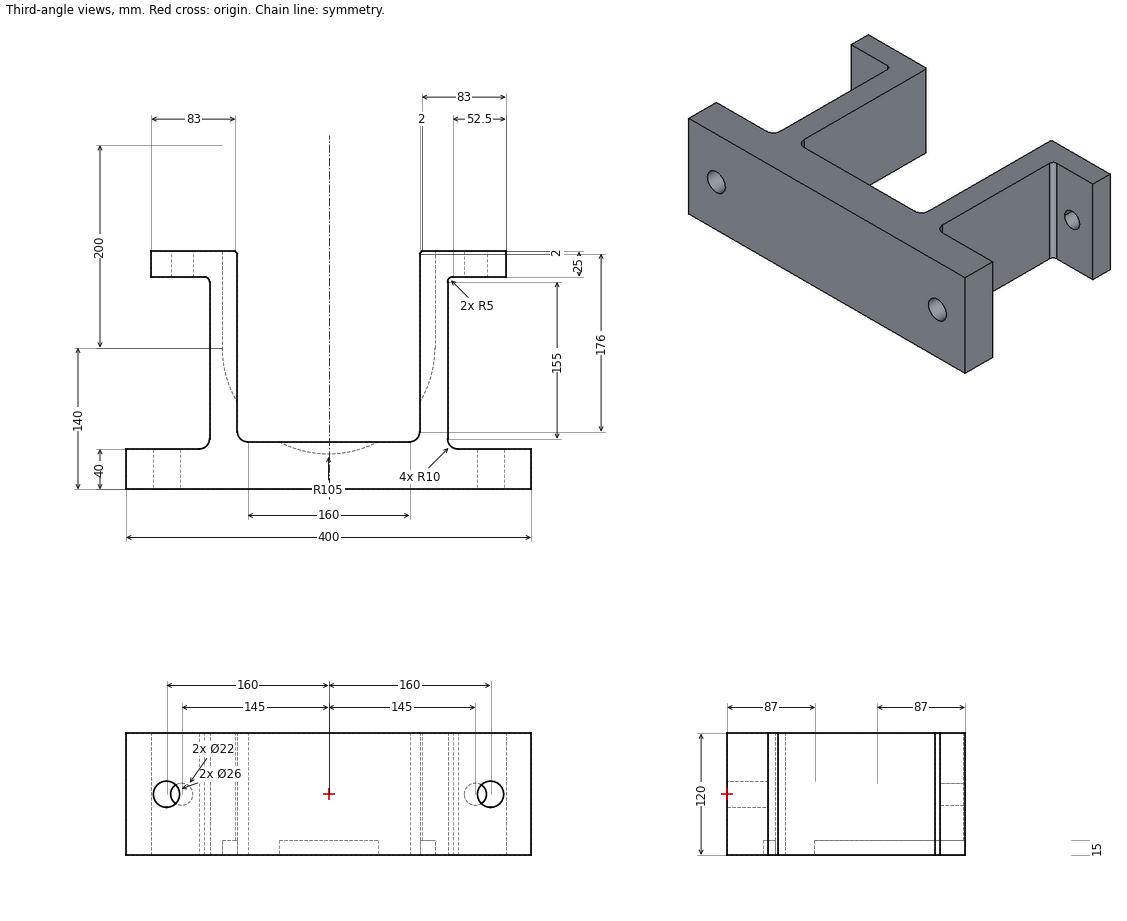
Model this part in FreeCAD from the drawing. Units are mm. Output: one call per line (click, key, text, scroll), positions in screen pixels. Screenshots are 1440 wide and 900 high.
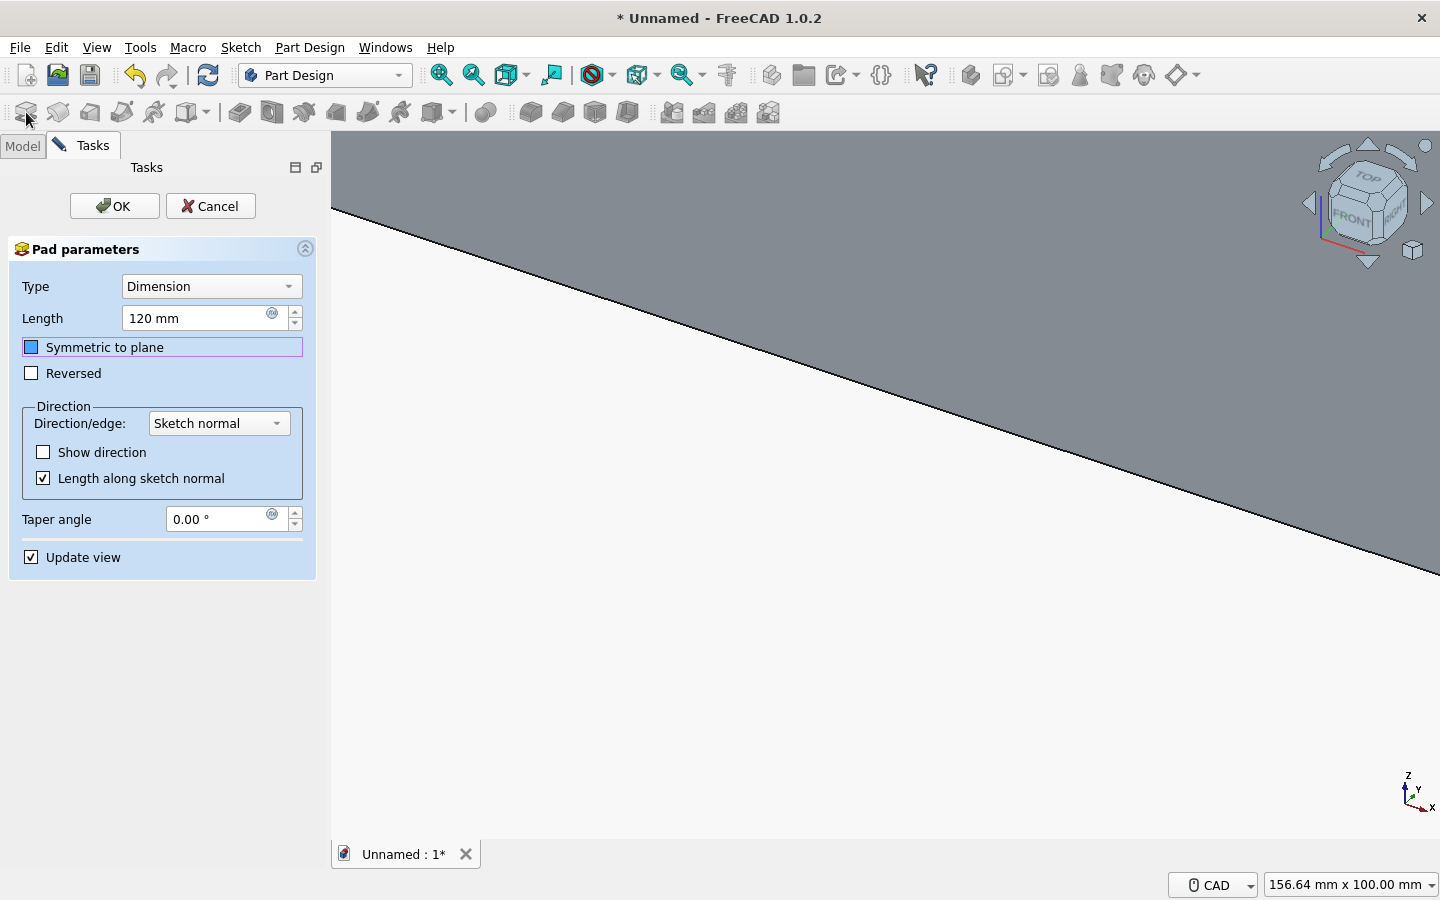
click(30, 347)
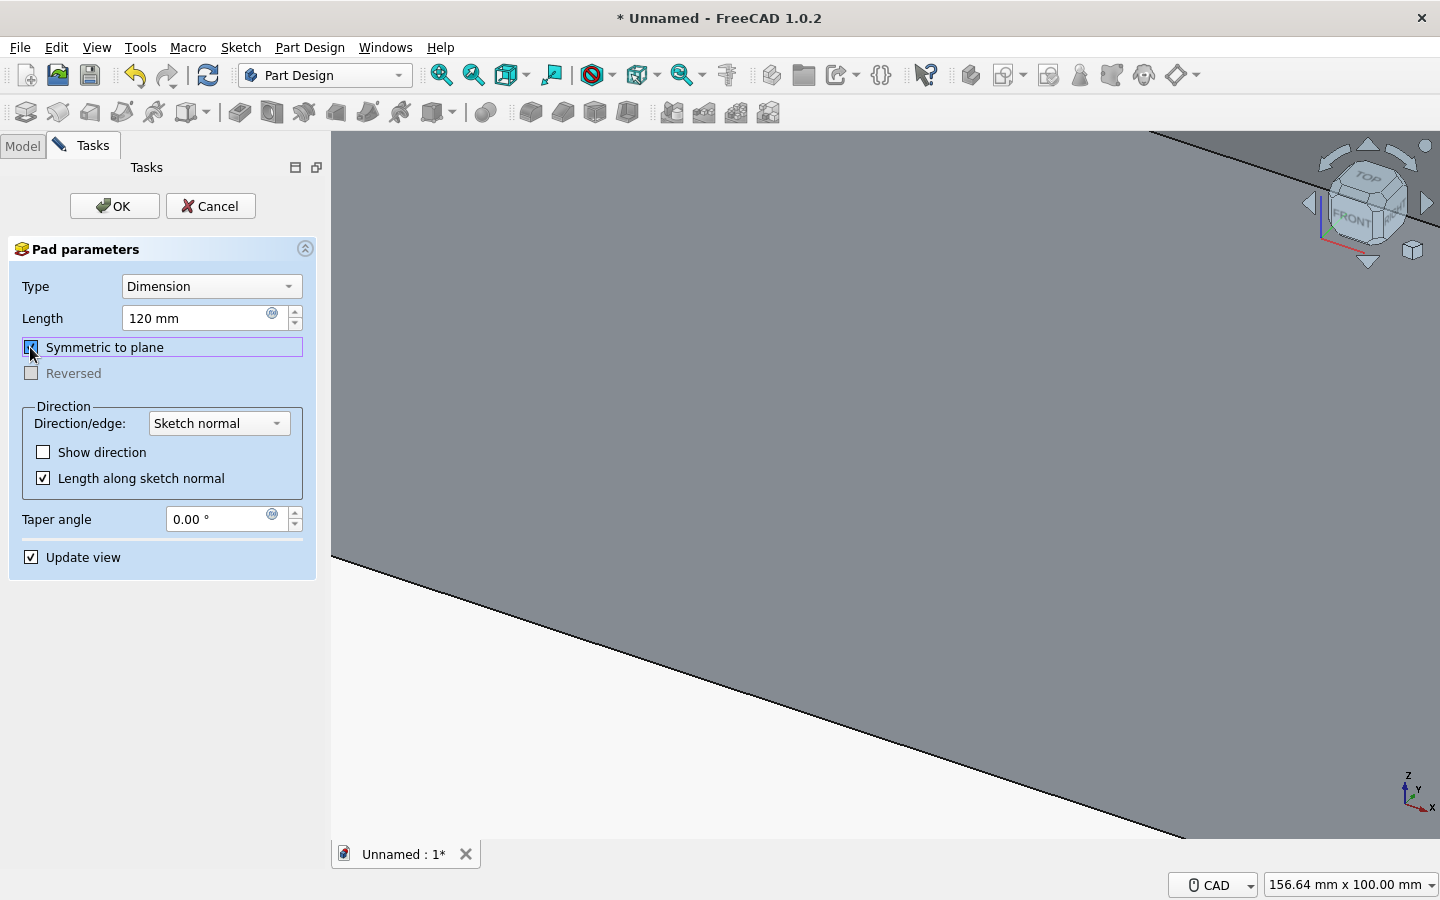
click(115, 206)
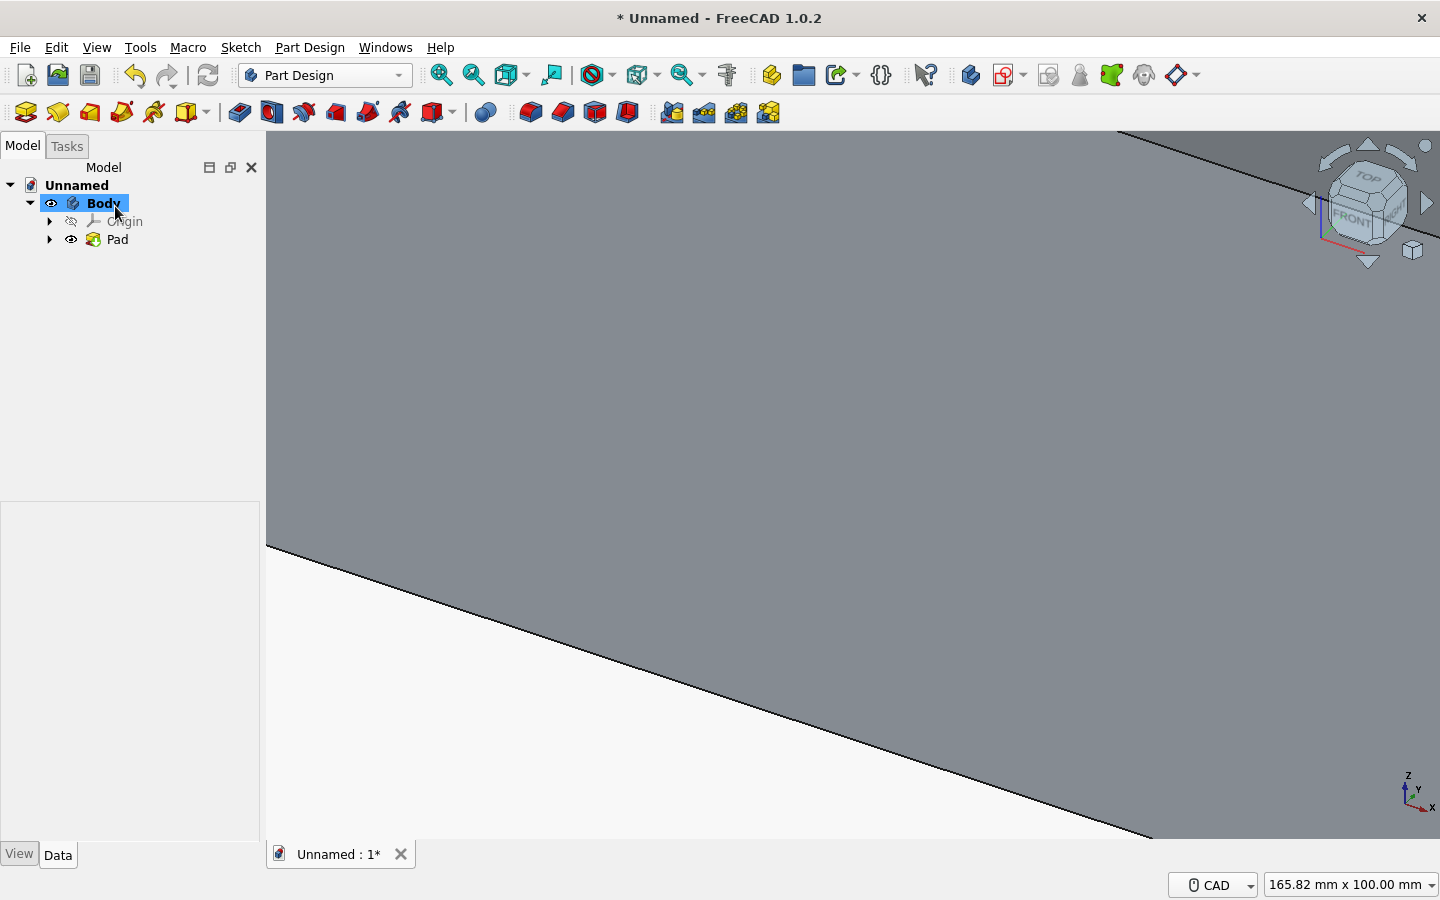
click(442, 76)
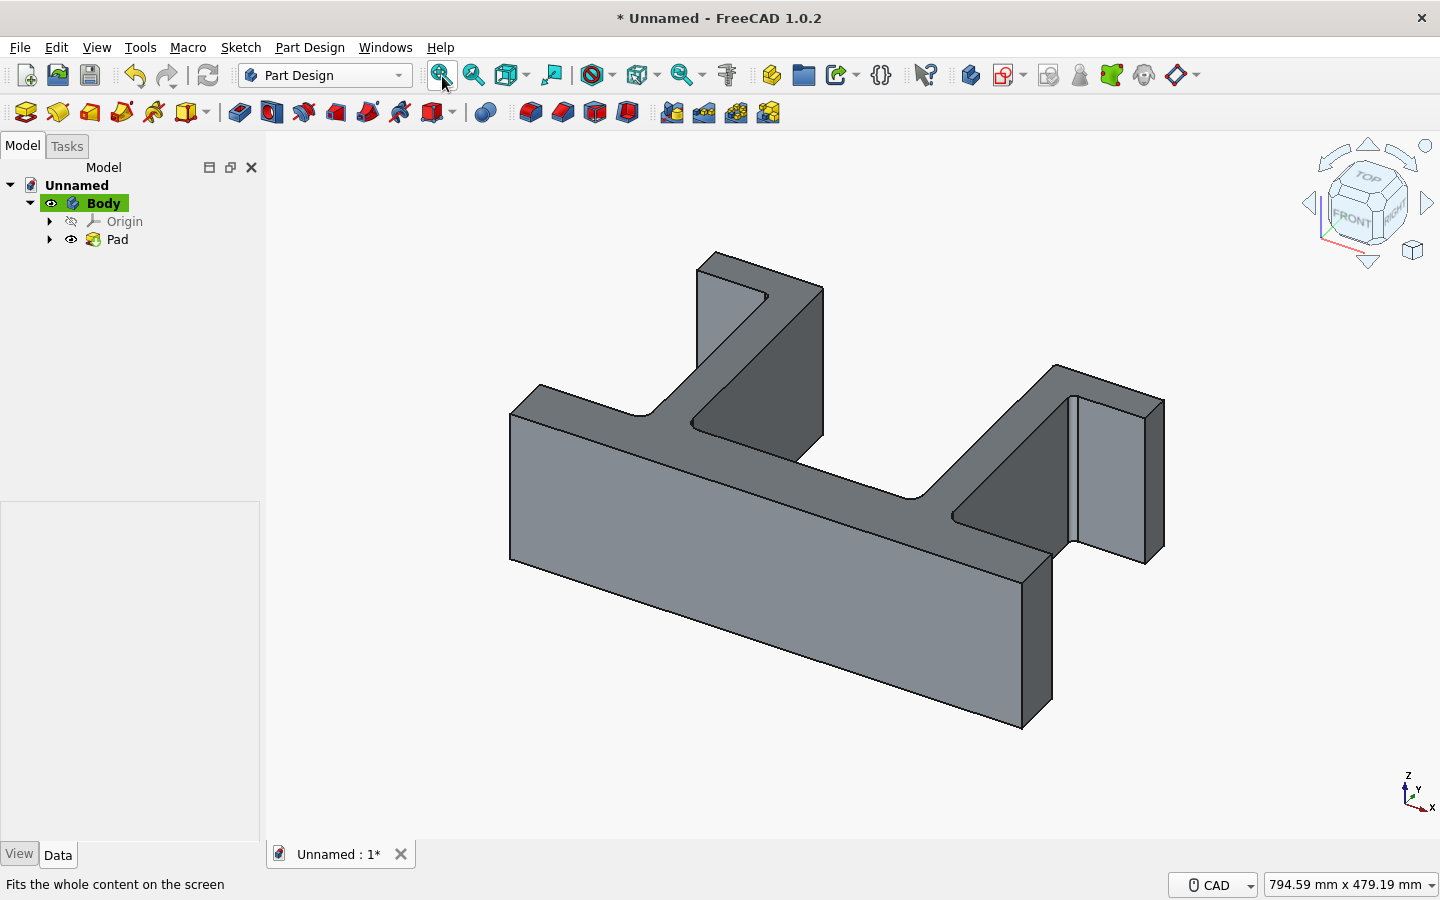
click(1004, 76)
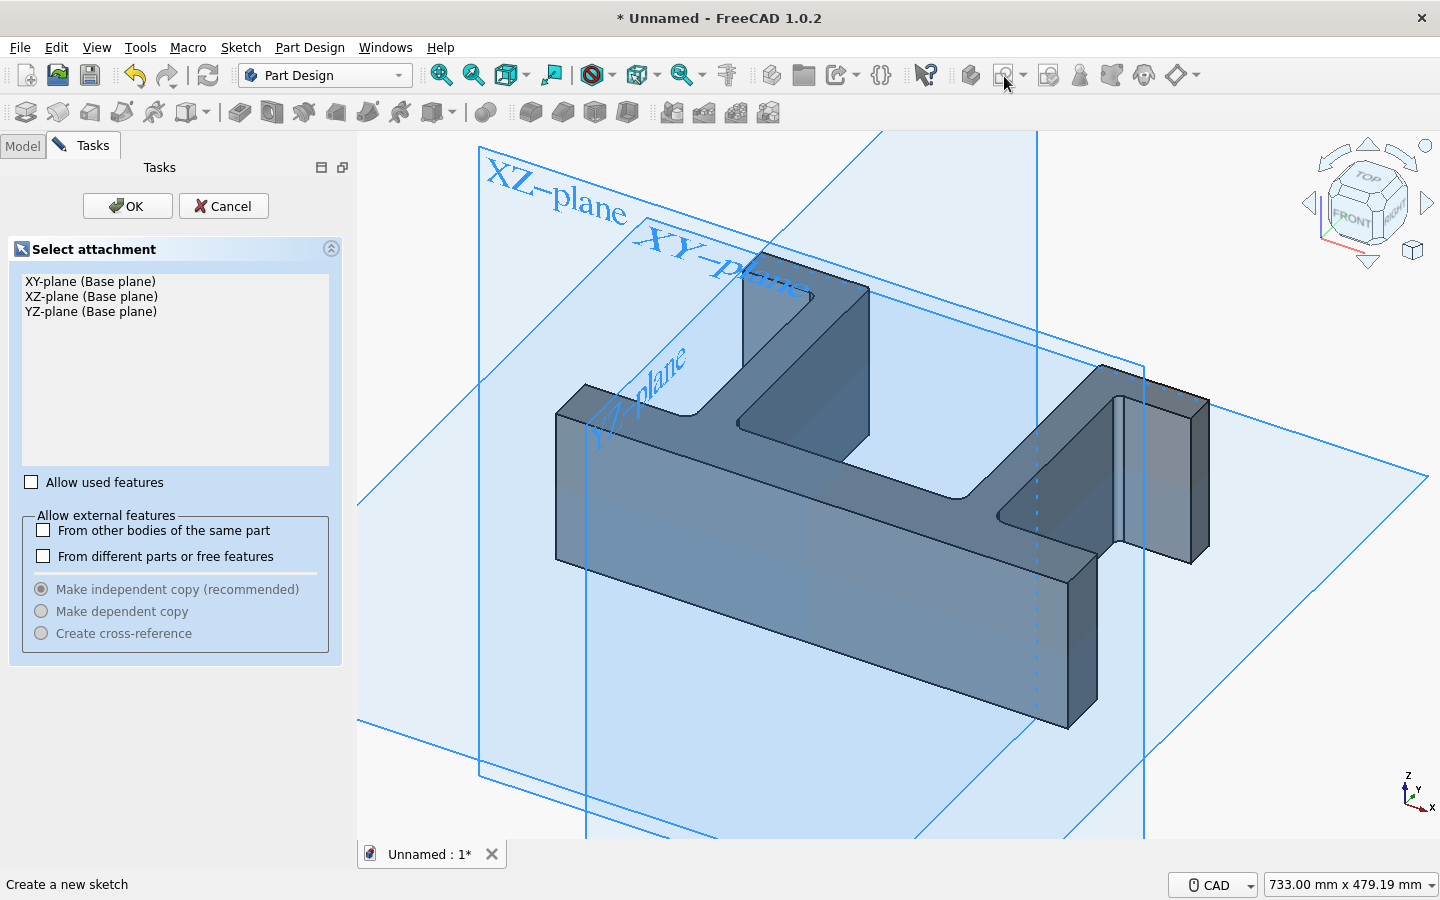
click(82, 296)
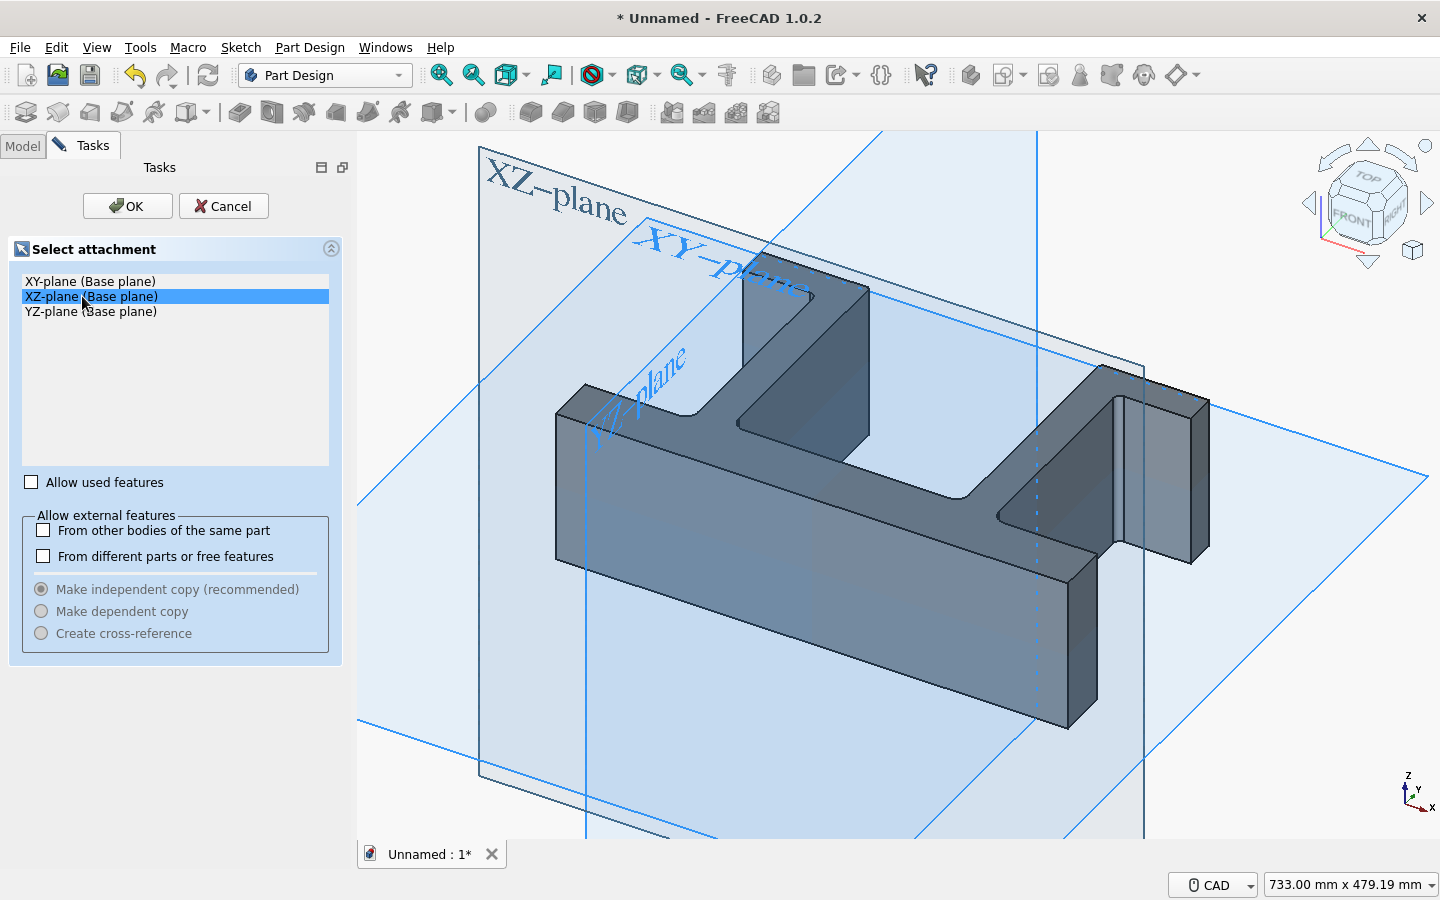
click(128, 206)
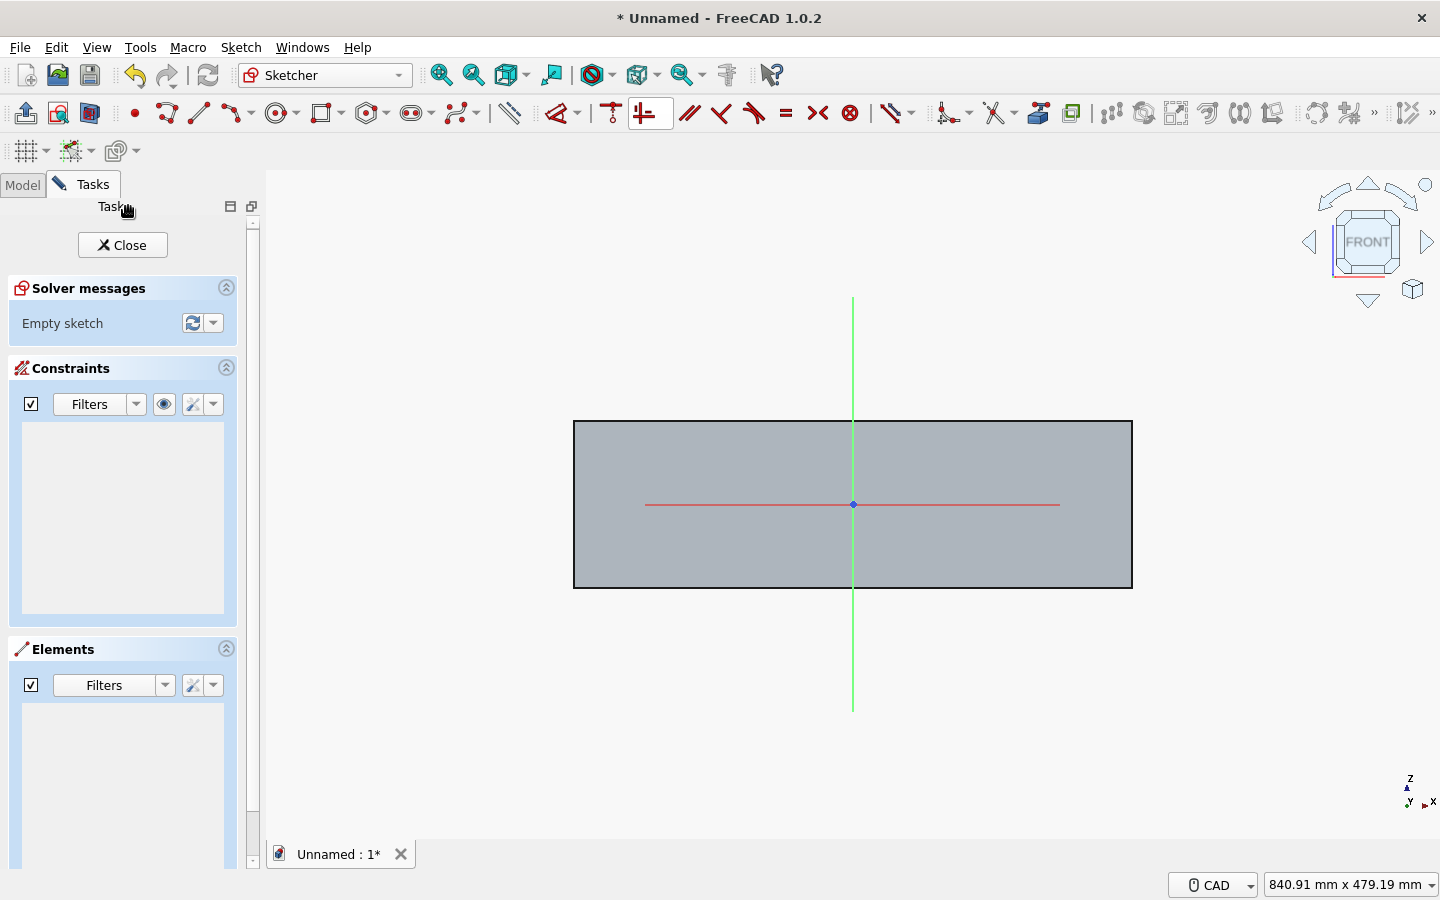
scroll(992, 505, up, 2)